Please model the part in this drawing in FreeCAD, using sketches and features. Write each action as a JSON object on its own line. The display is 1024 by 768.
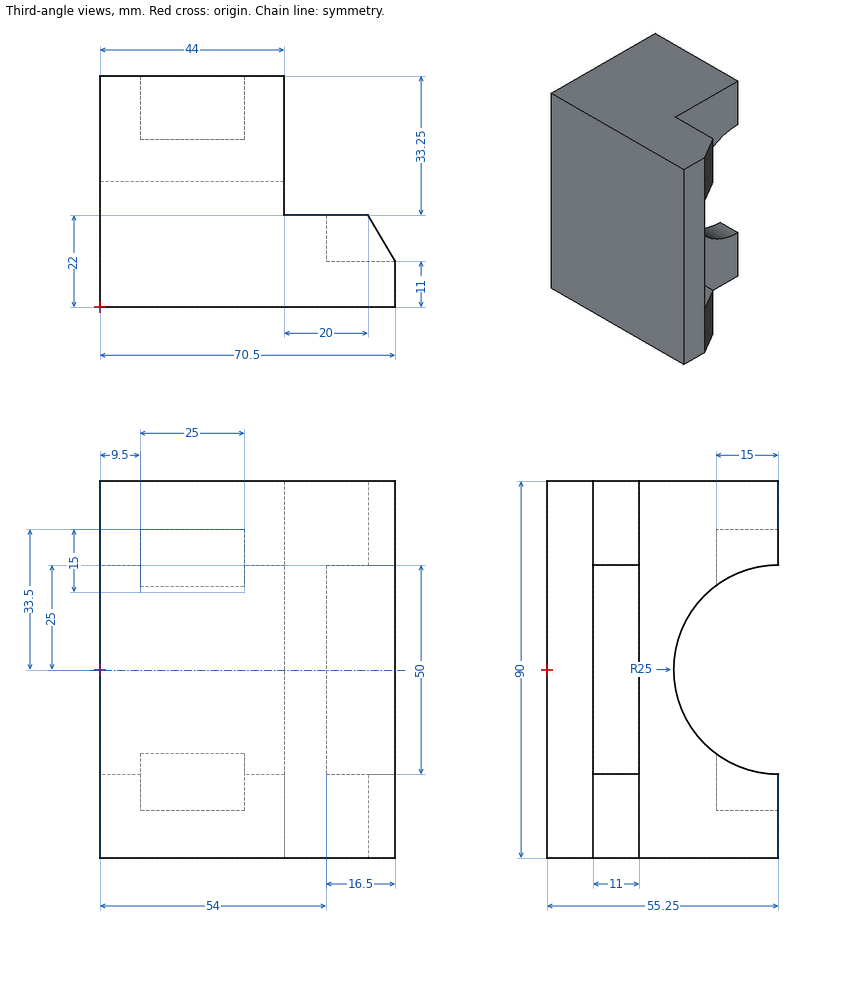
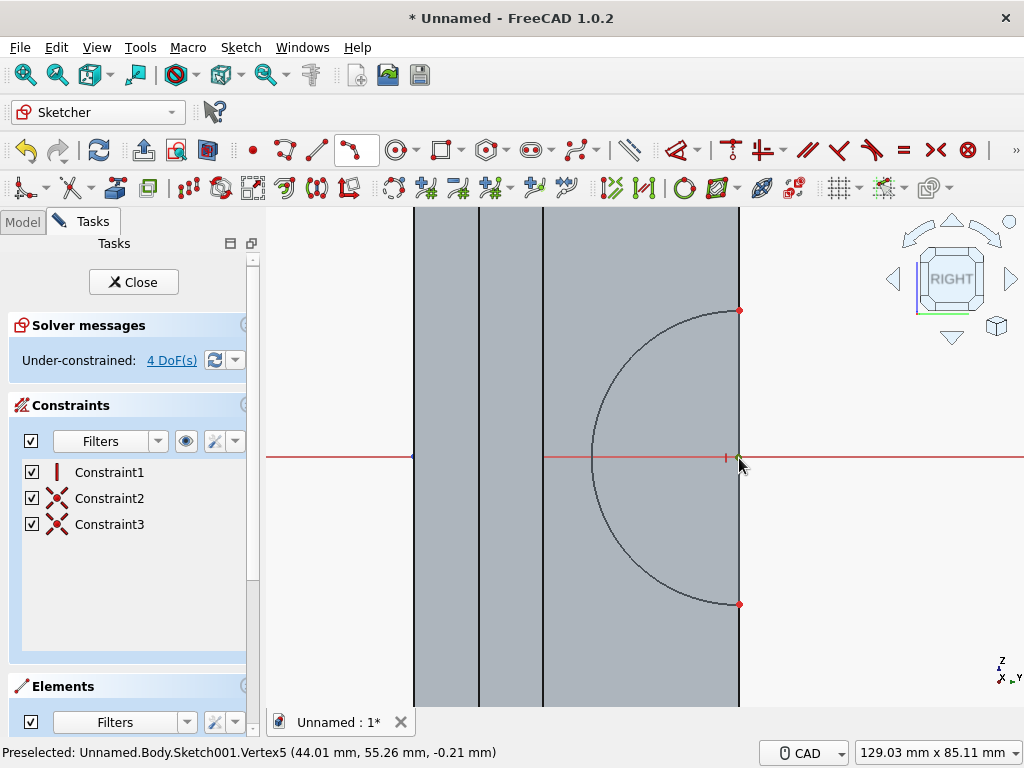
{"action": "left_click", "coordinate": [334, 457]}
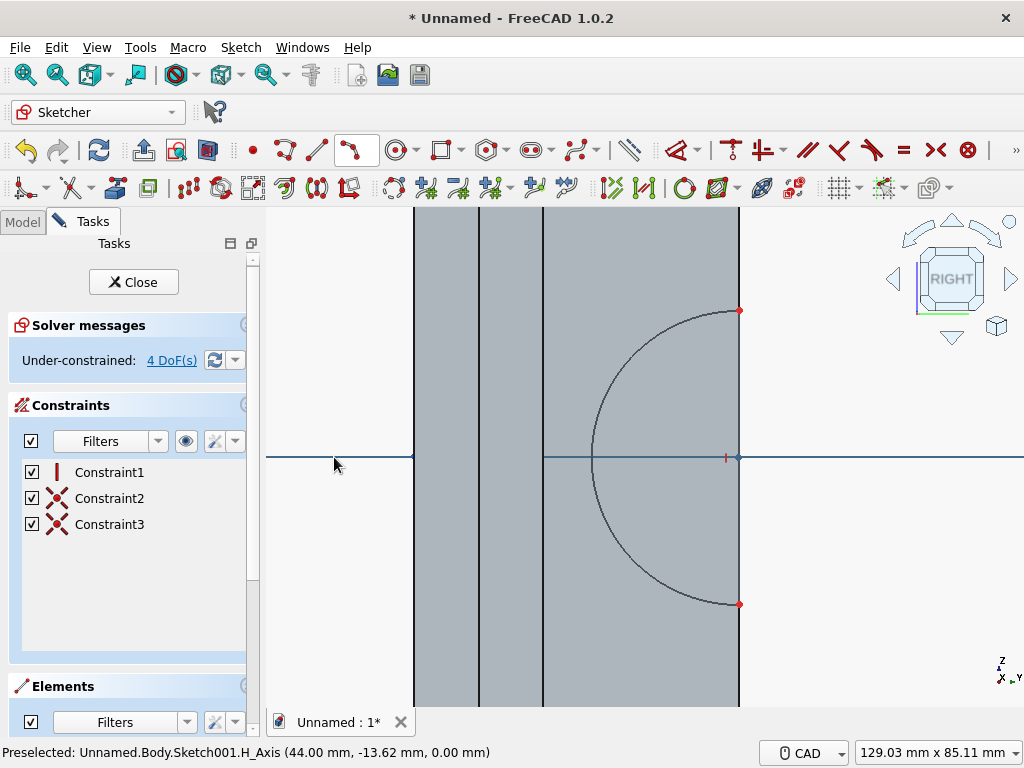
{"action": "left_click", "coordinate": [732, 150]}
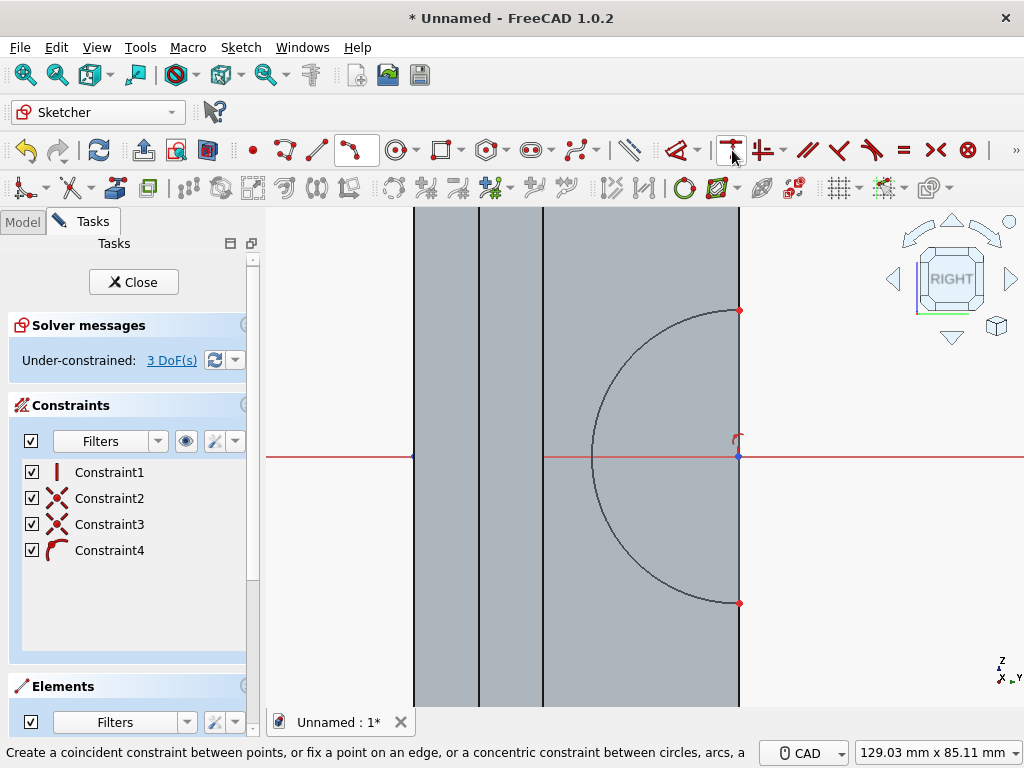
{"action": "left_click", "coordinate": [676, 150]}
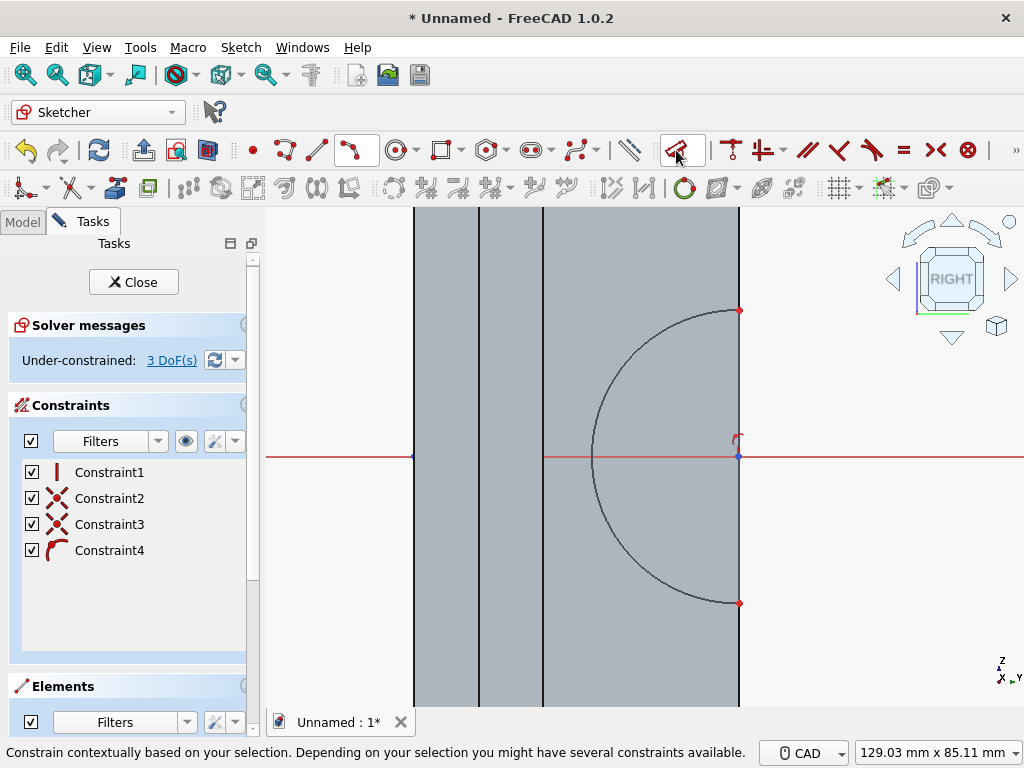
{"action": "left_click", "coordinate": [620, 370]}
{"action": "left_click", "coordinate": [594, 351]}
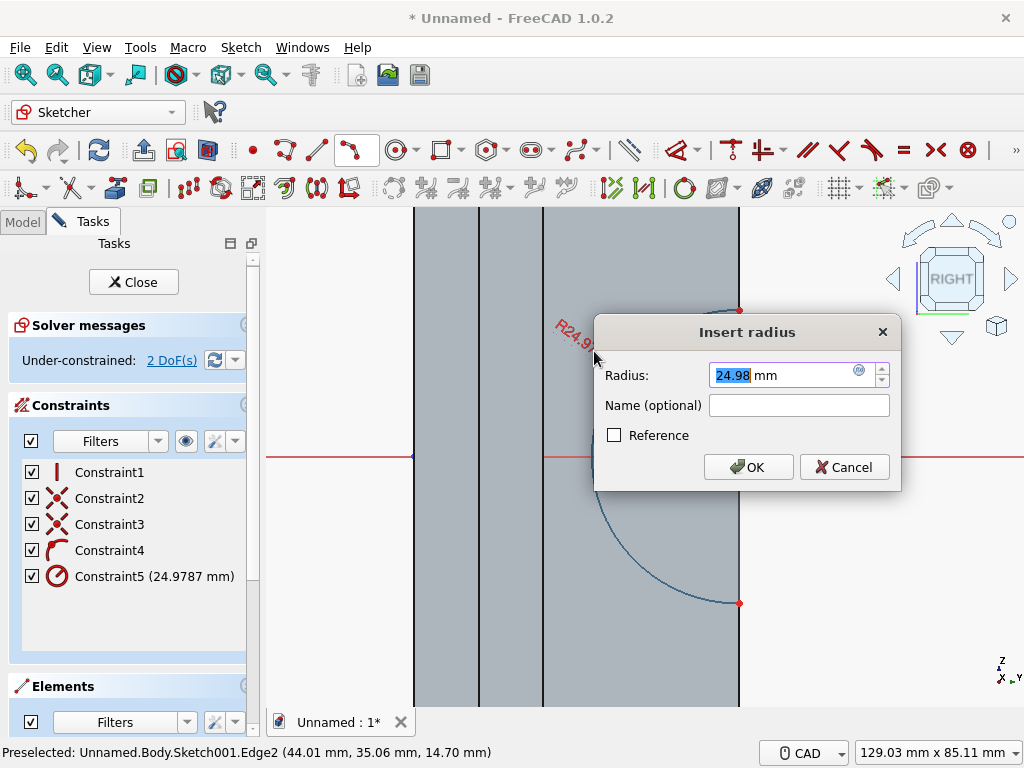
{"action": "type", "text": "25"}
{"action": "key", "text": "Return"}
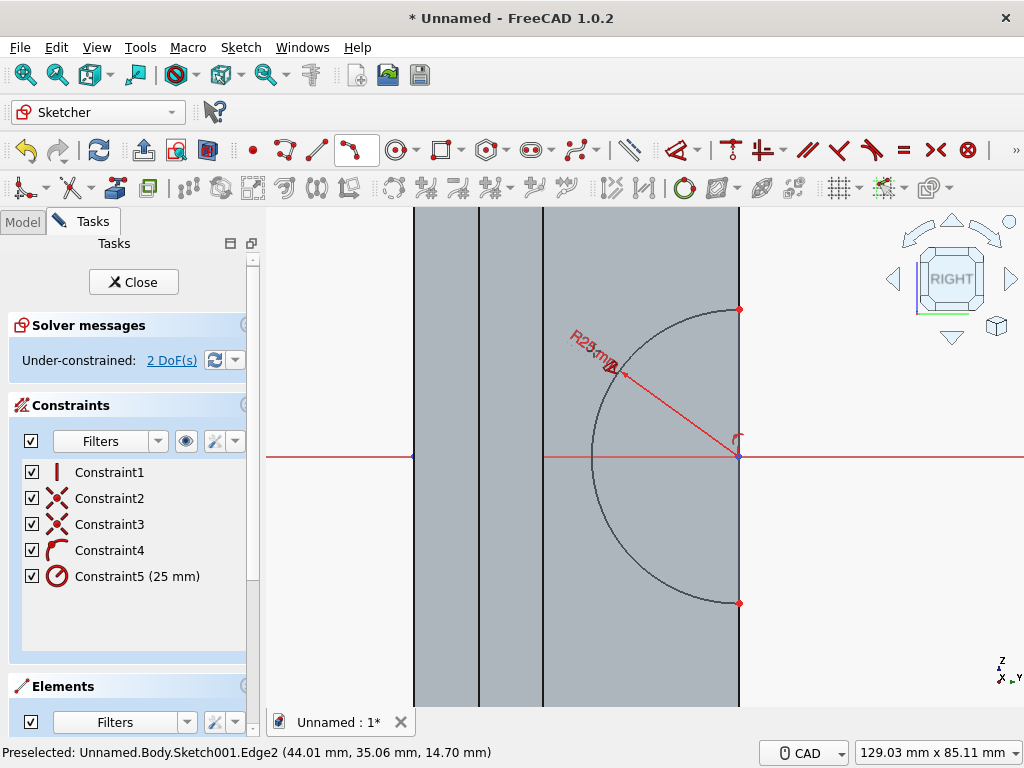
{"action": "left_click", "coordinate": [739, 604]}
{"action": "left_click", "coordinate": [577, 638]}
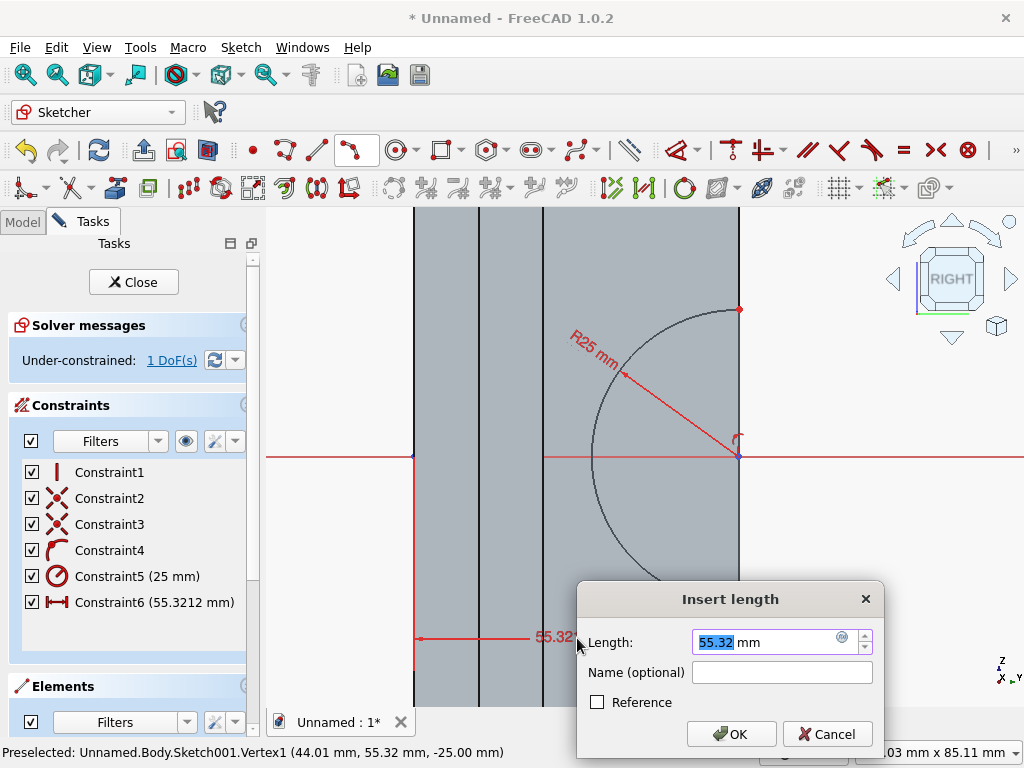
{"action": "type", "text": "55.25"}
{"action": "key", "text": "Return"}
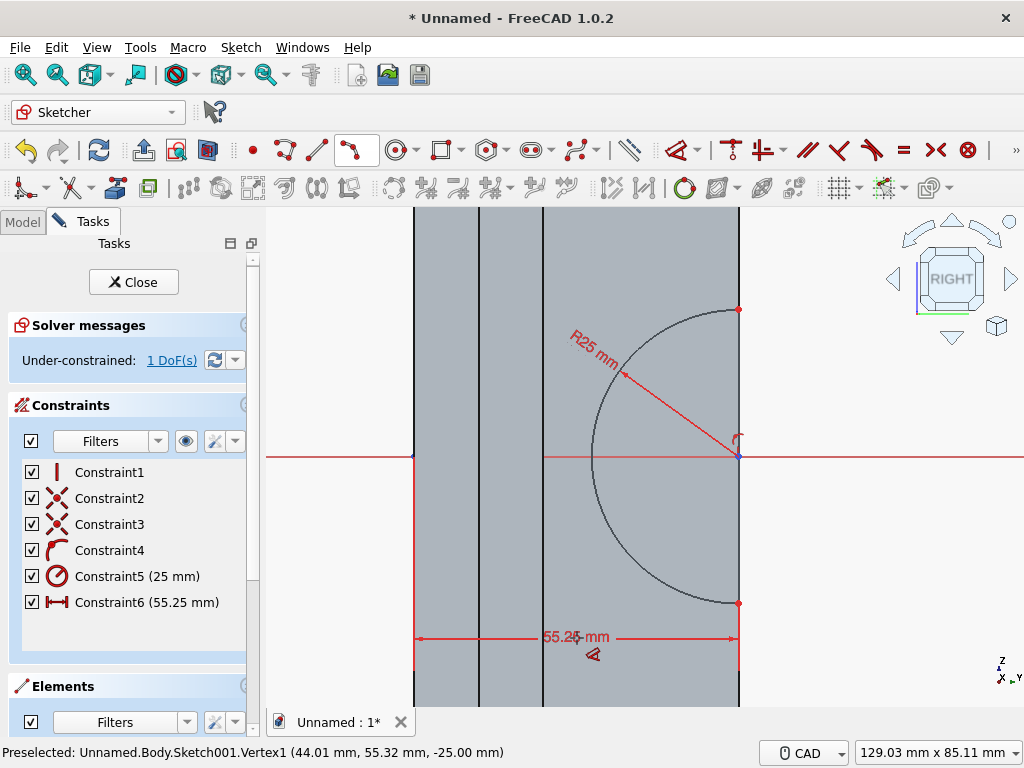
{"action": "left_click", "coordinate": [739, 457]}
{"action": "left_click", "coordinate": [576, 491]}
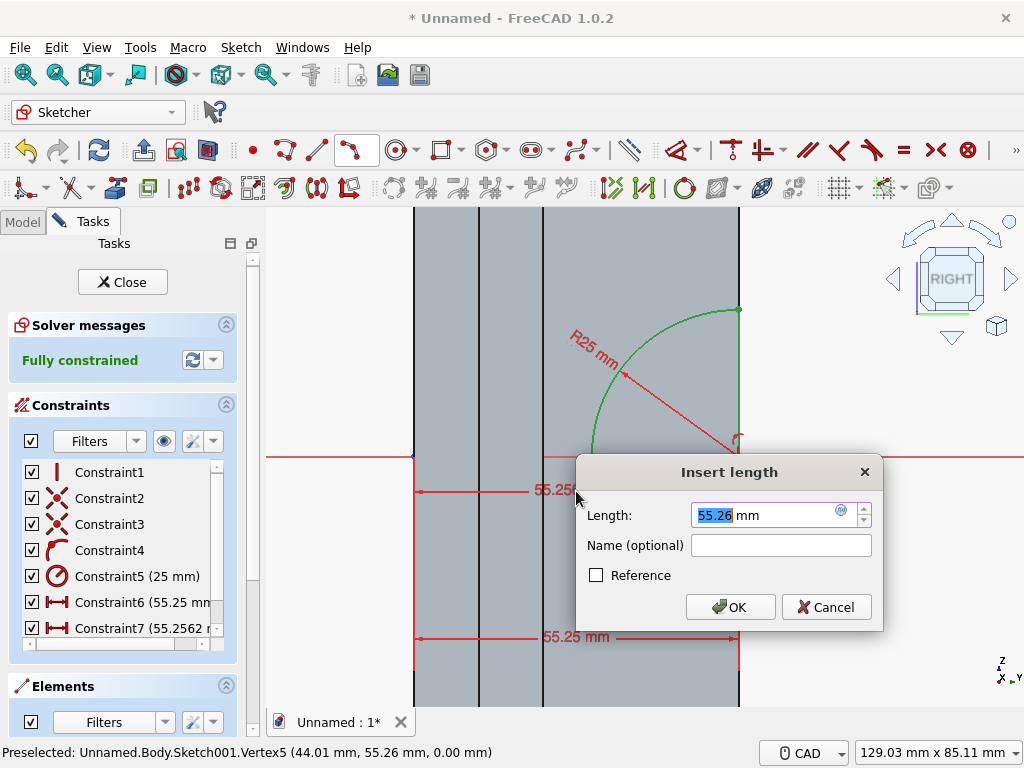
{"action": "type", "text": "55.25"}
{"action": "key", "text": "Return"}
{"action": "key", "text": "Escape"}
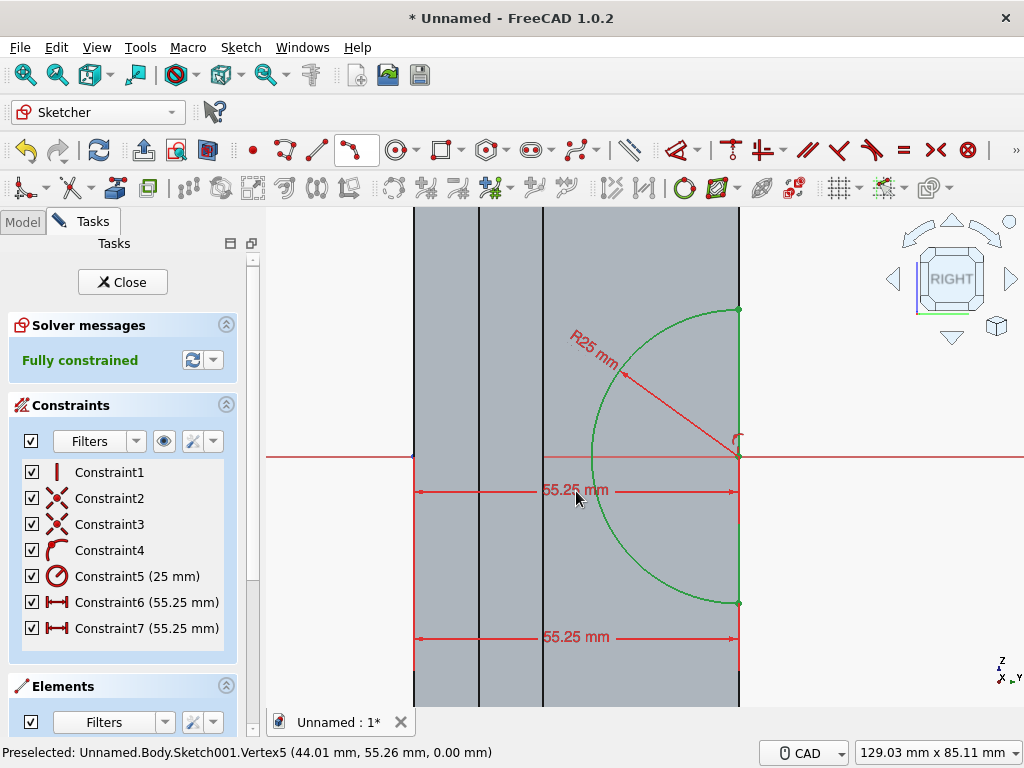
{"action": "left_click", "coordinate": [123, 282]}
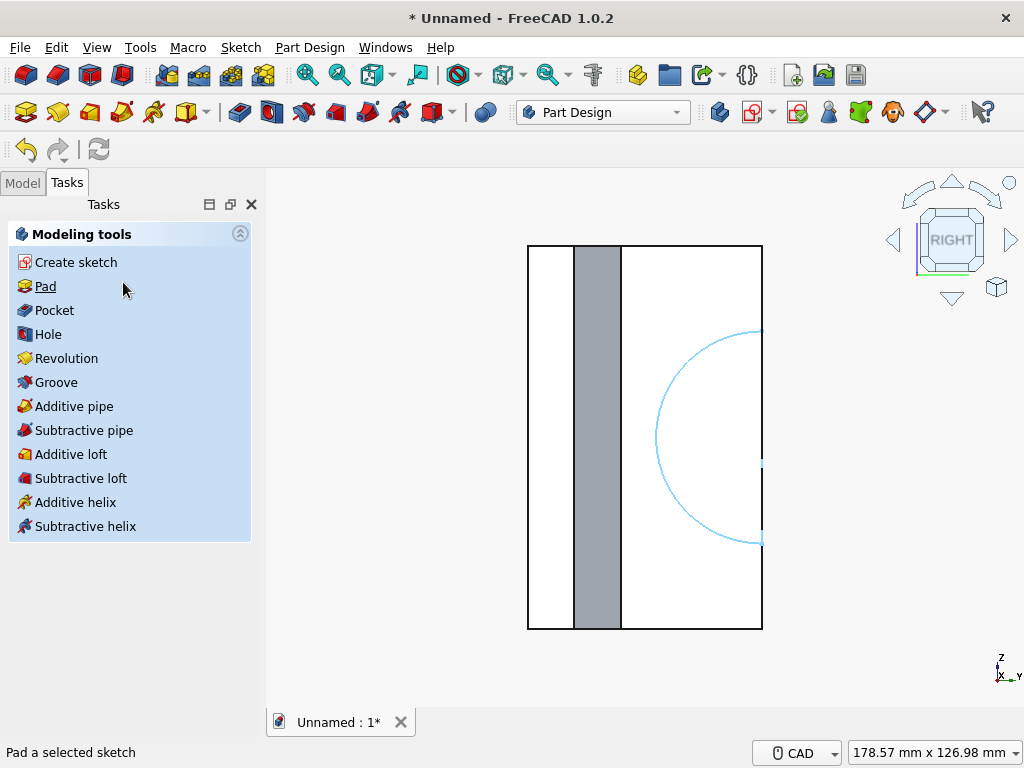
{"action": "left_click", "coordinate": [240, 112]}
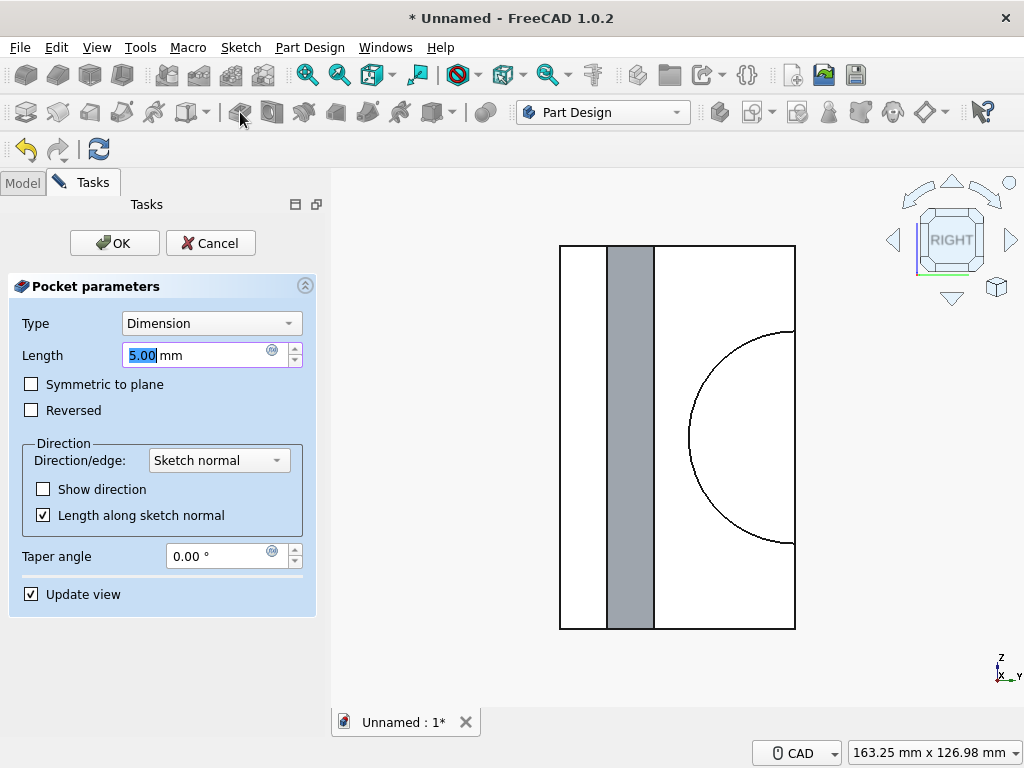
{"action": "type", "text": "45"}
{"action": "key", "text": "Tab"}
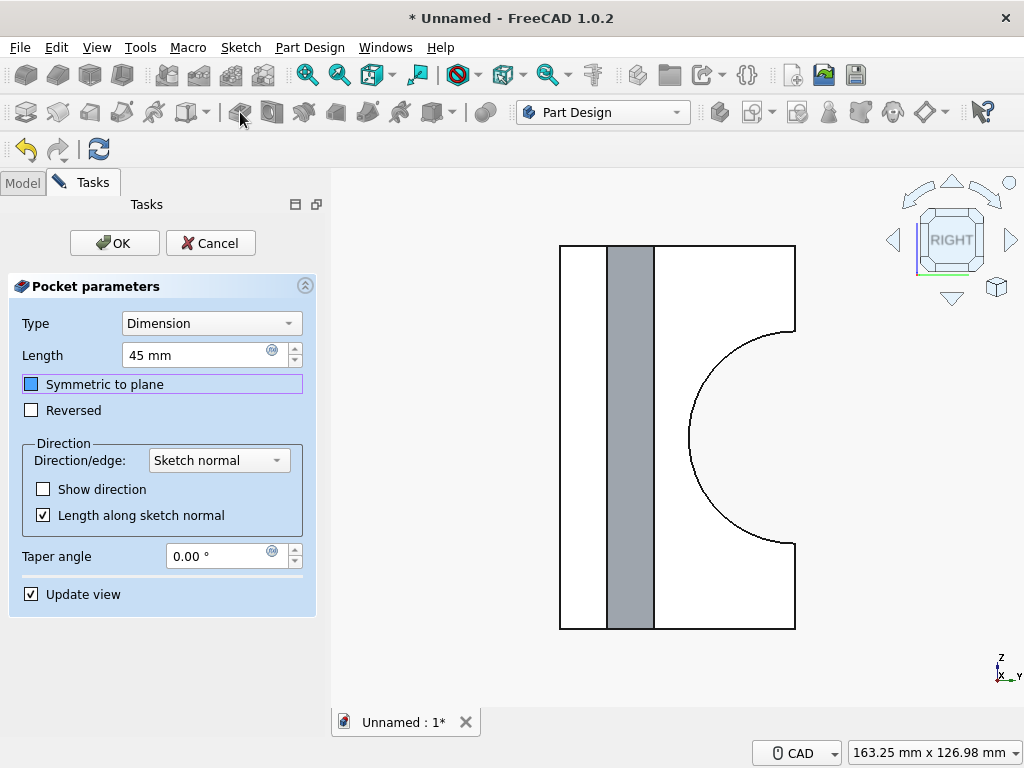
{"action": "left_click", "coordinate": [115, 243]}